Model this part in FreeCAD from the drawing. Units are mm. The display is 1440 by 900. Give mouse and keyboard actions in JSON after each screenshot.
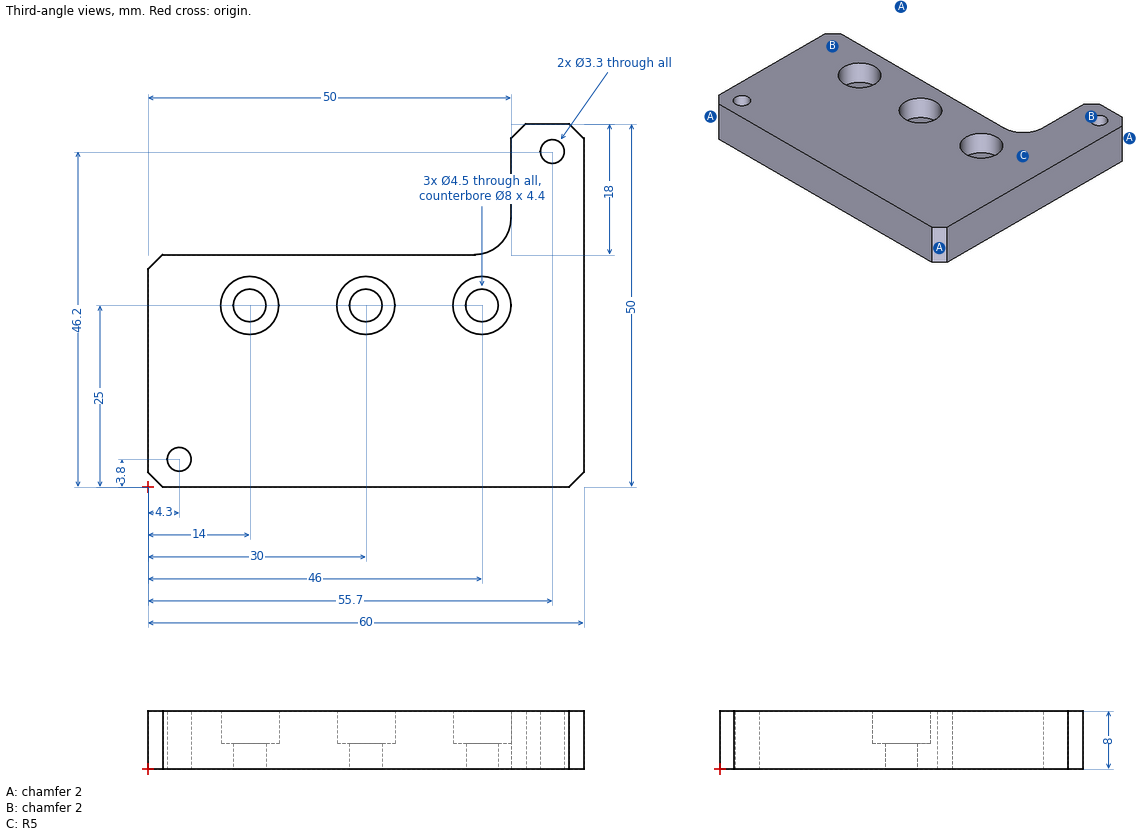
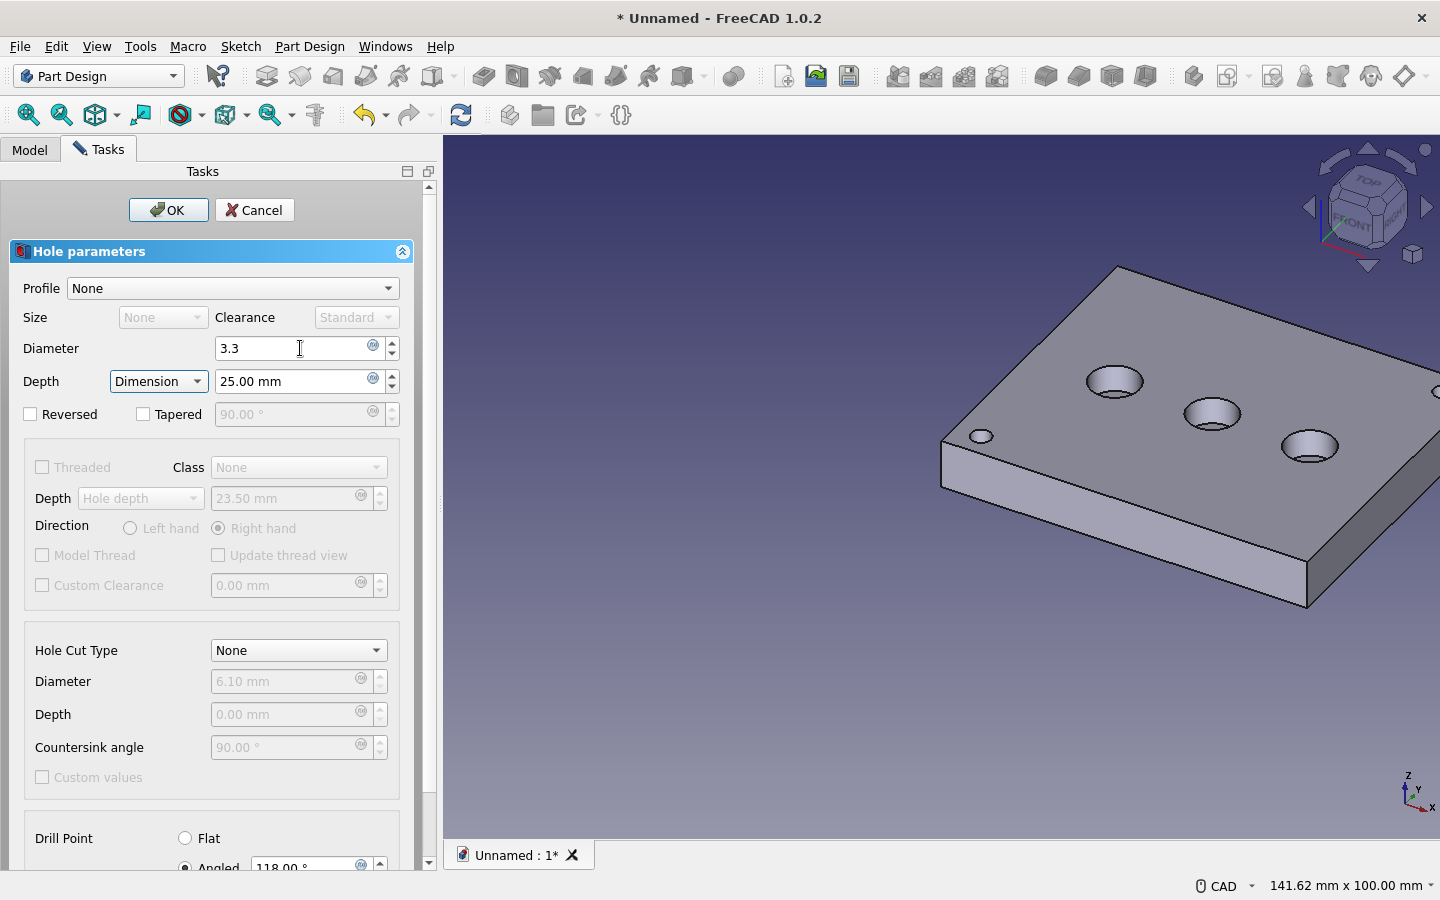
{"action": "left_click", "coordinate": [160, 382]}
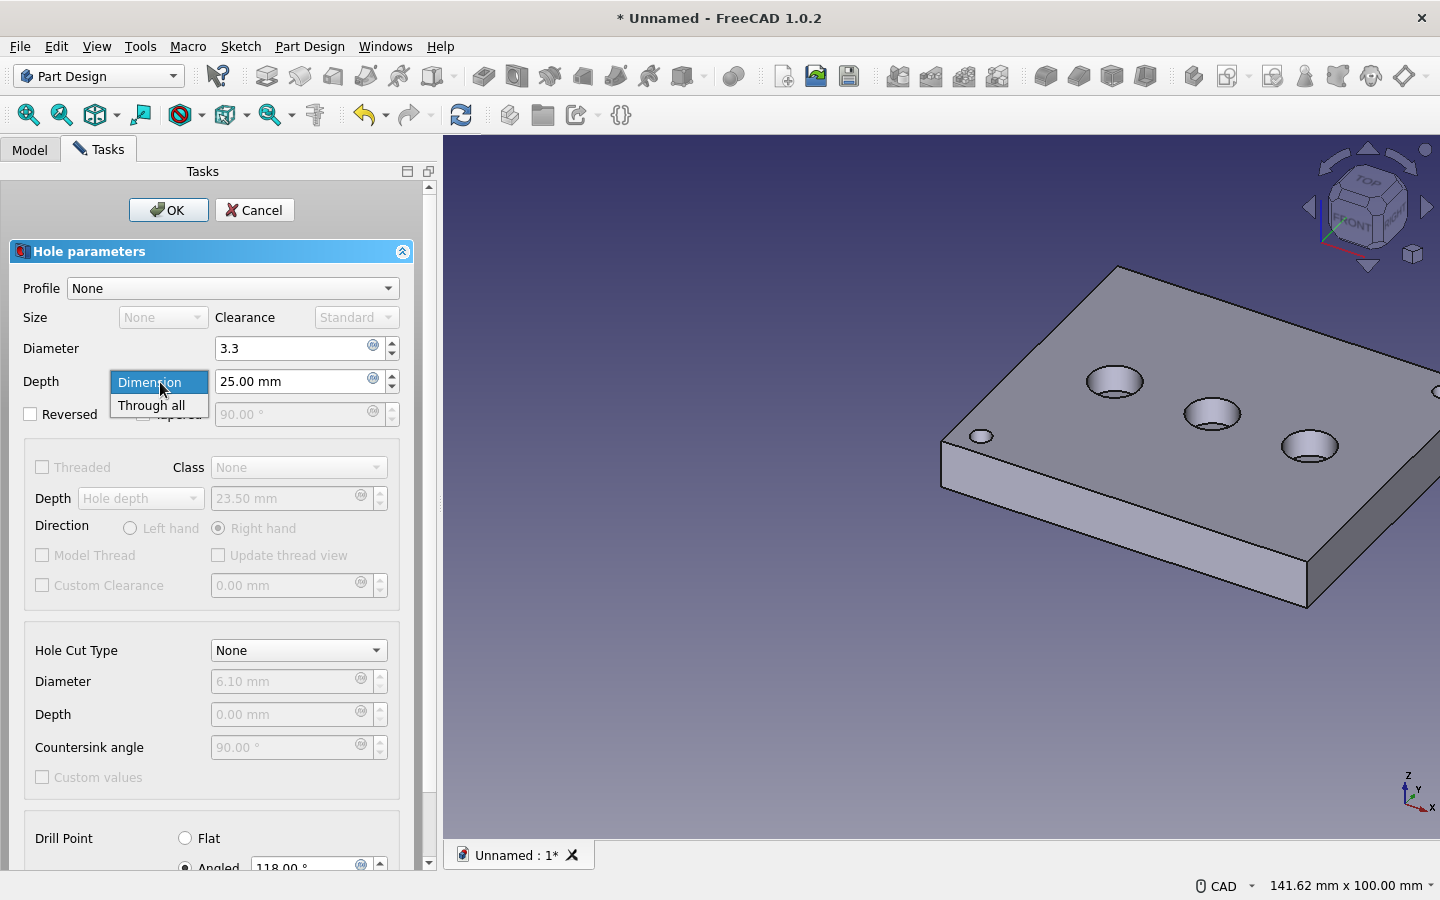
{"action": "left_click", "coordinate": [158, 406]}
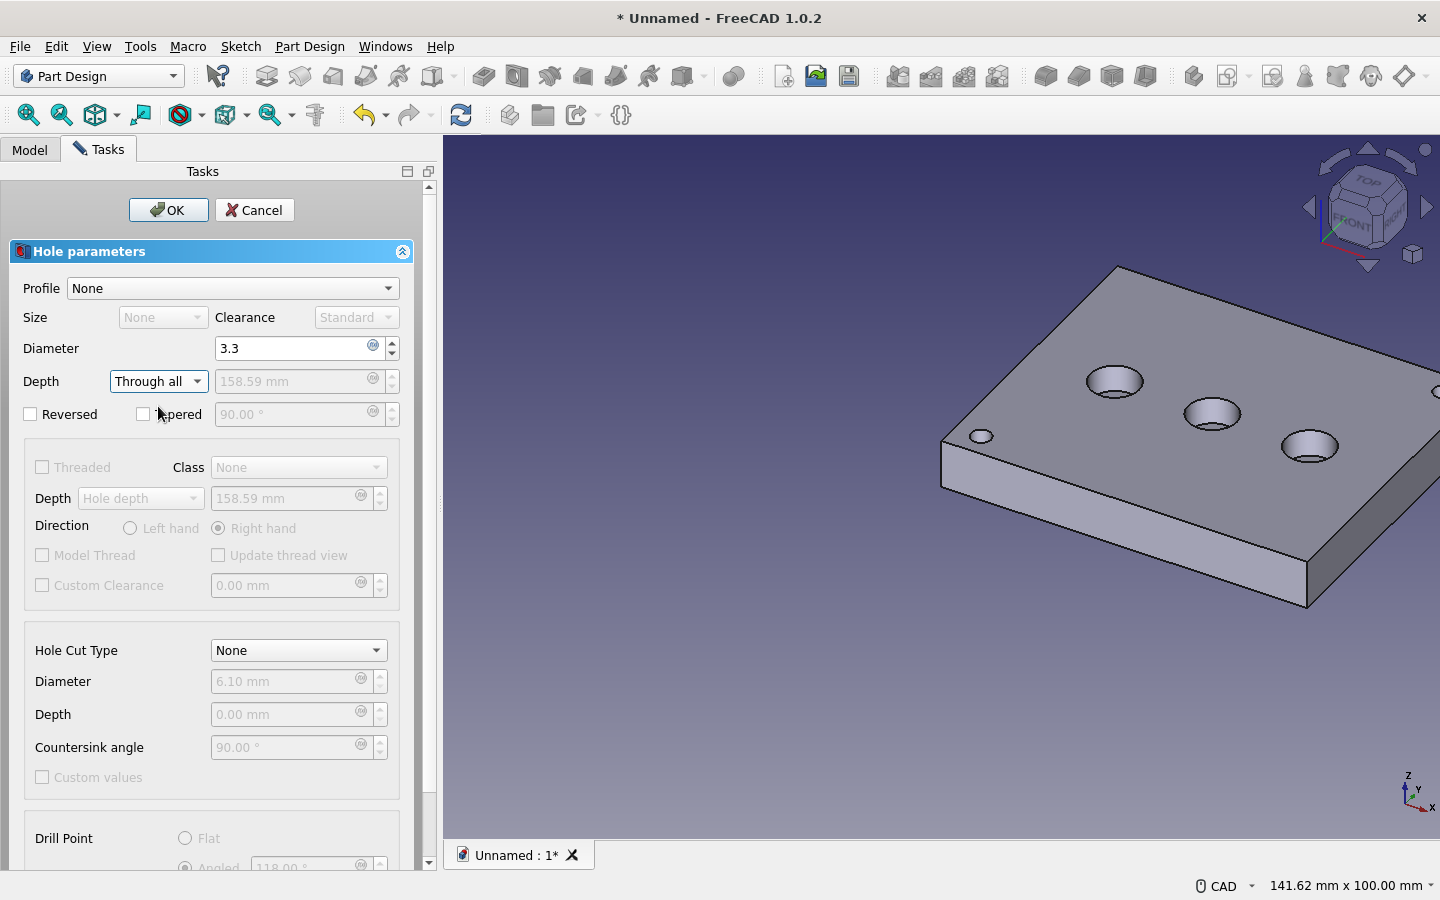
{"action": "left_click", "coordinate": [169, 210]}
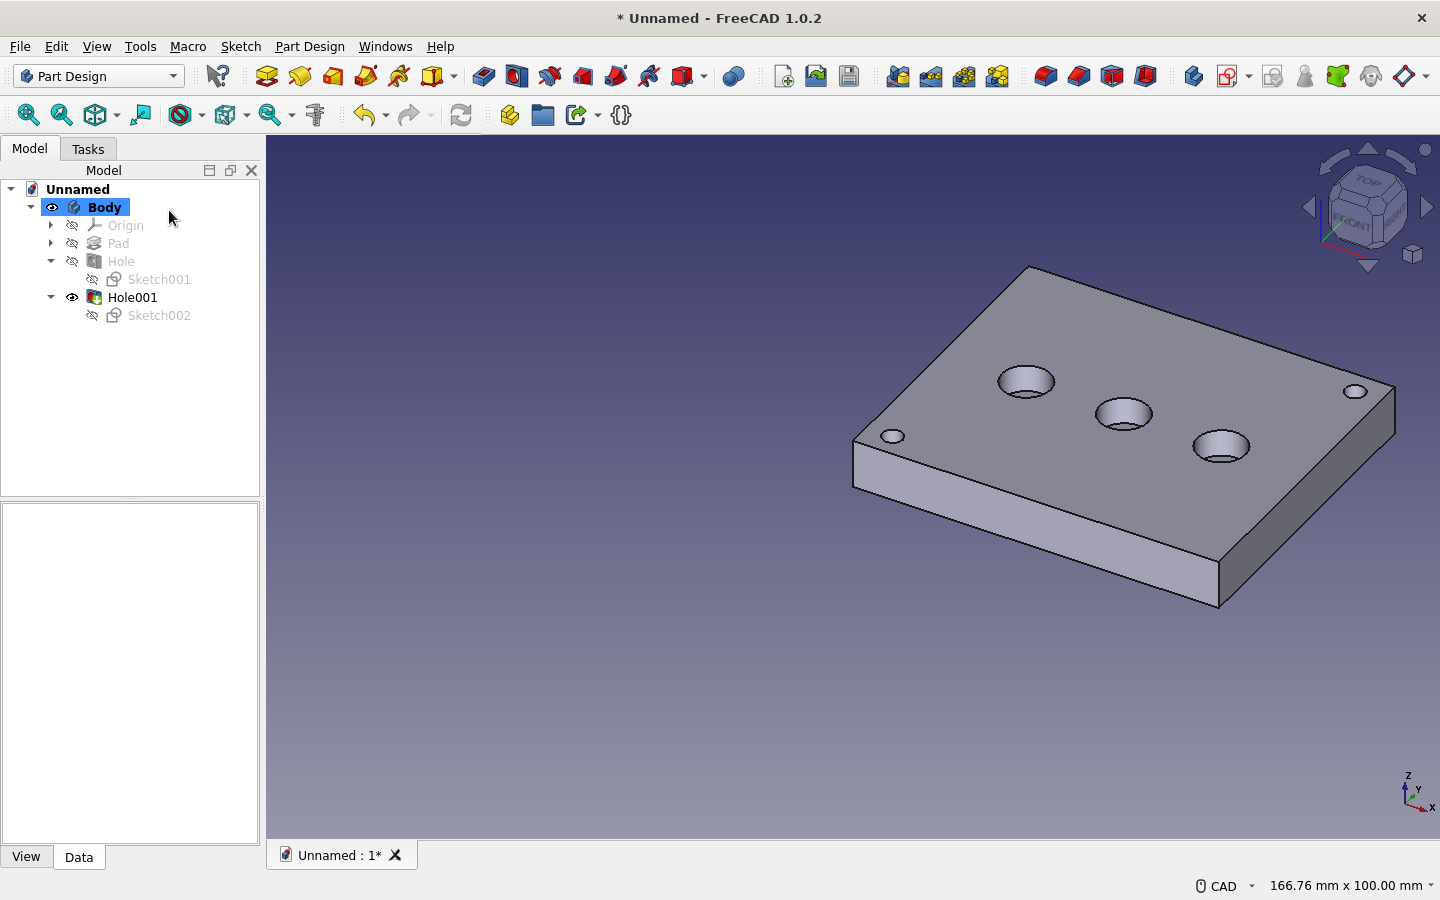
{"action": "left_click", "coordinate": [1219, 584]}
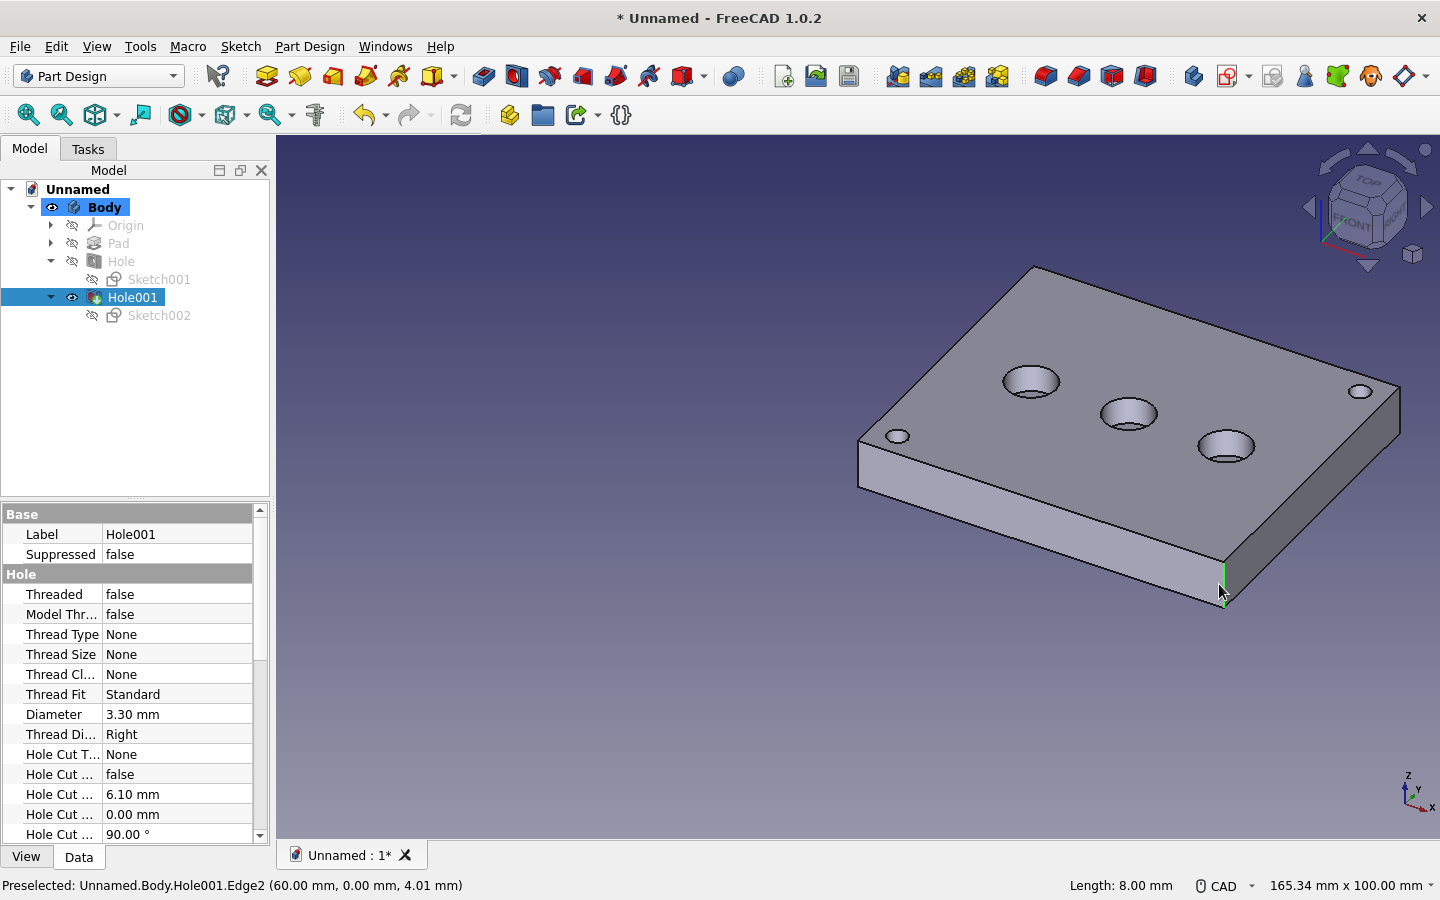
{"action": "key", "text": "0"}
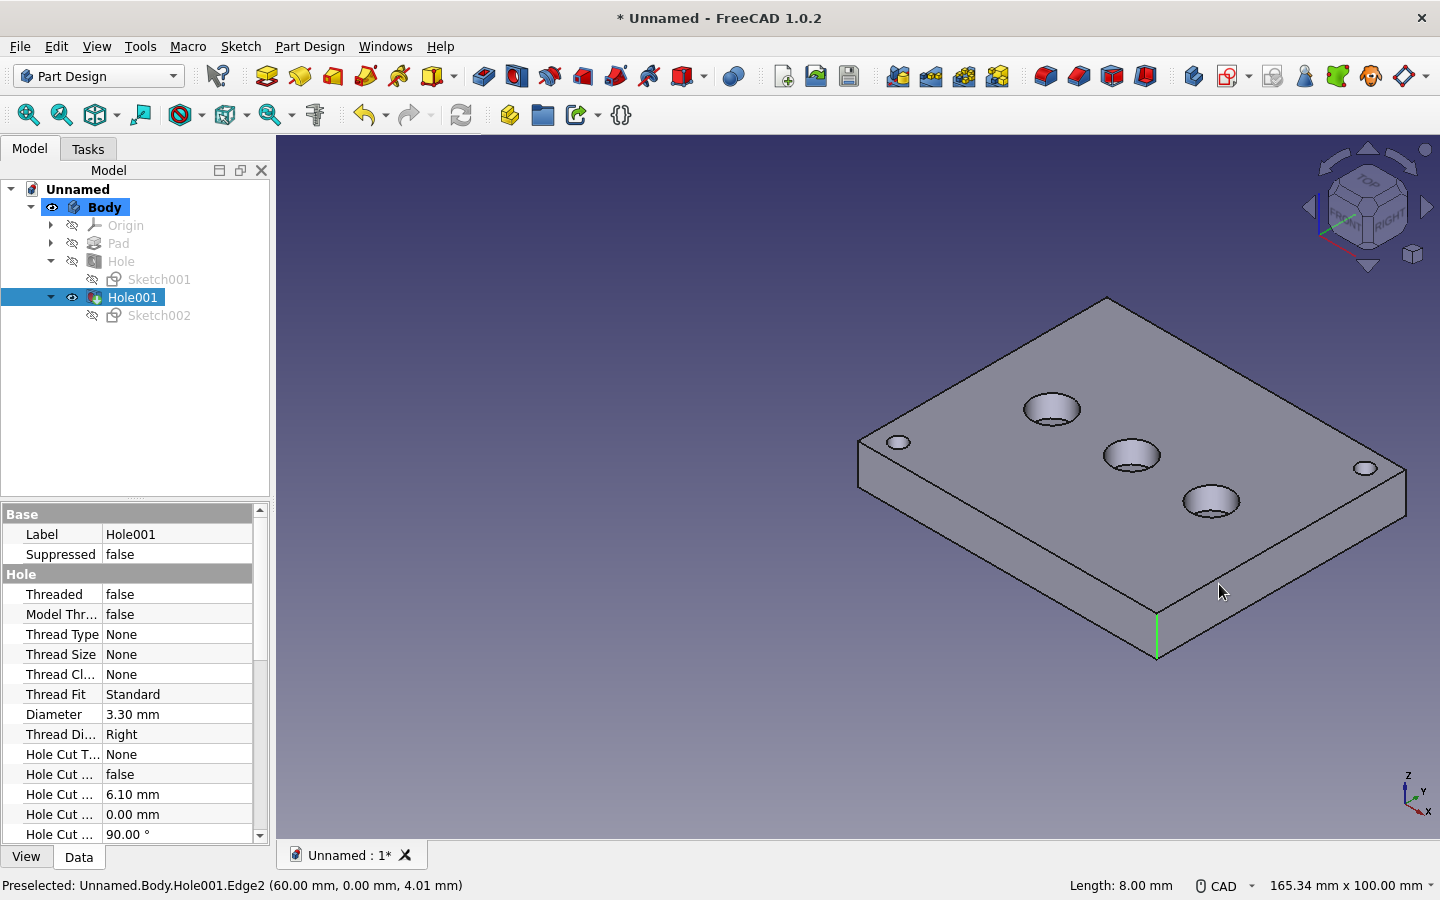
{"action": "key", "text": "2"}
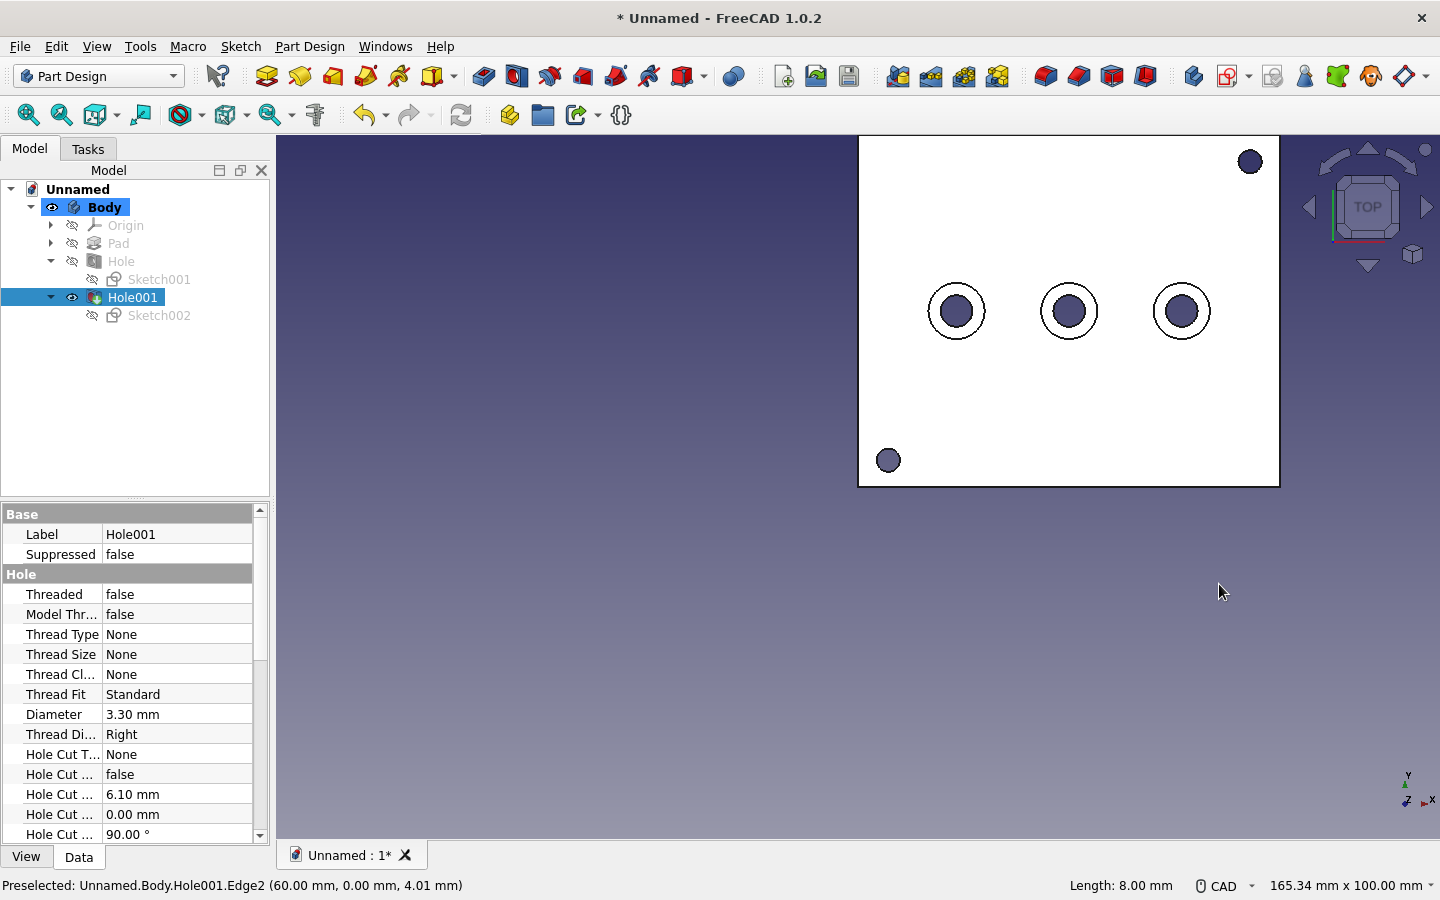
{"action": "left_click", "coordinate": [29, 116]}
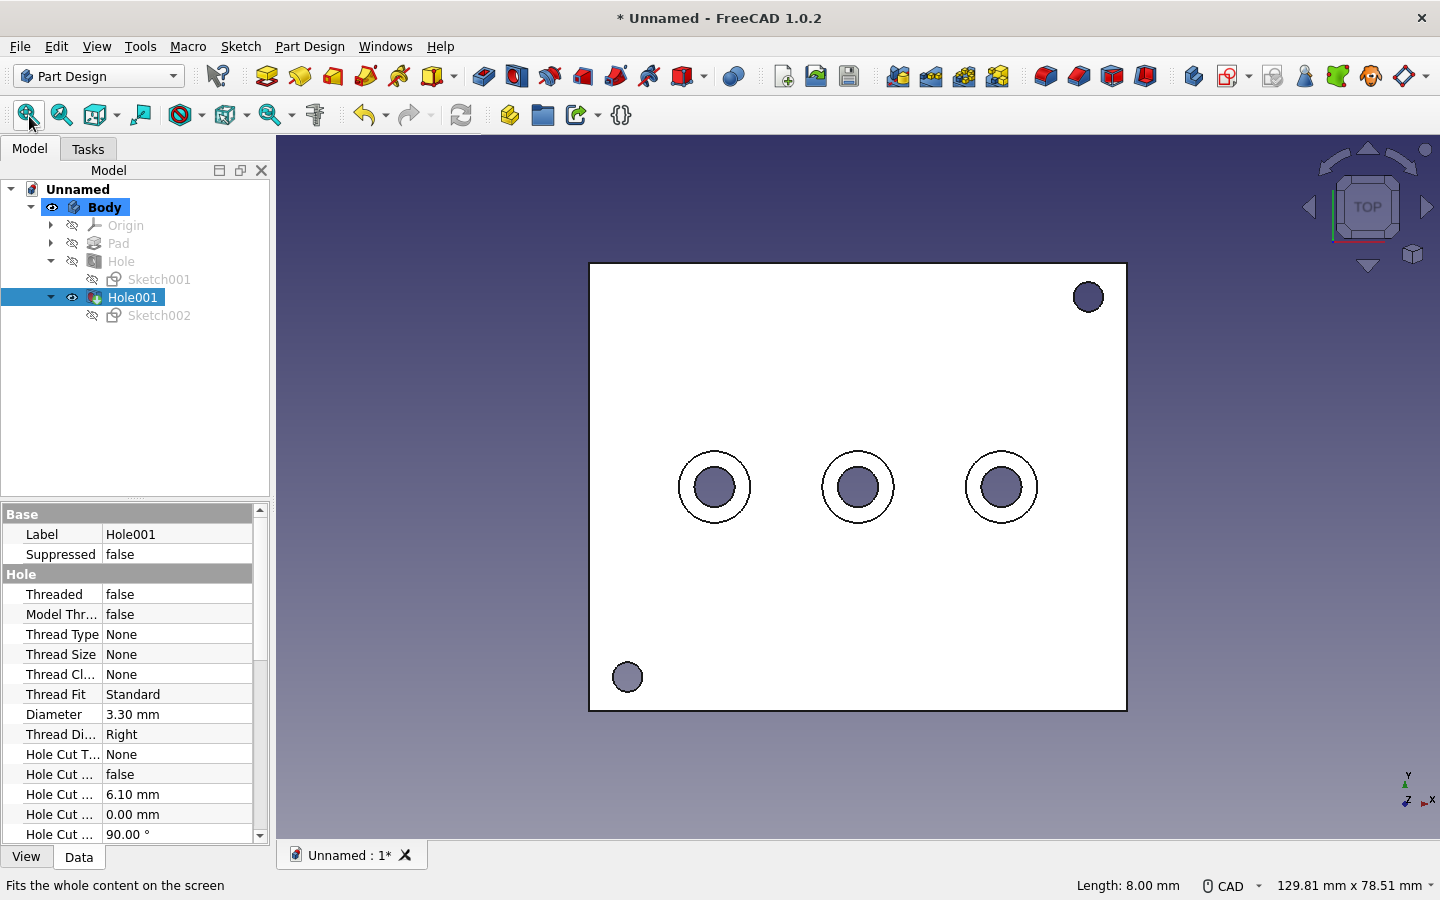
{"action": "key", "text": "1"}